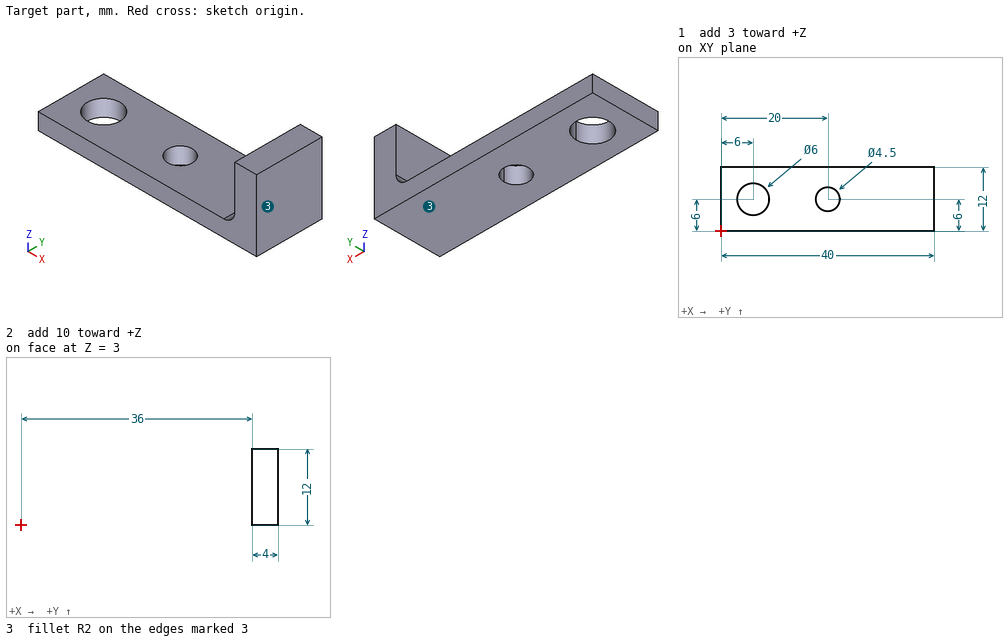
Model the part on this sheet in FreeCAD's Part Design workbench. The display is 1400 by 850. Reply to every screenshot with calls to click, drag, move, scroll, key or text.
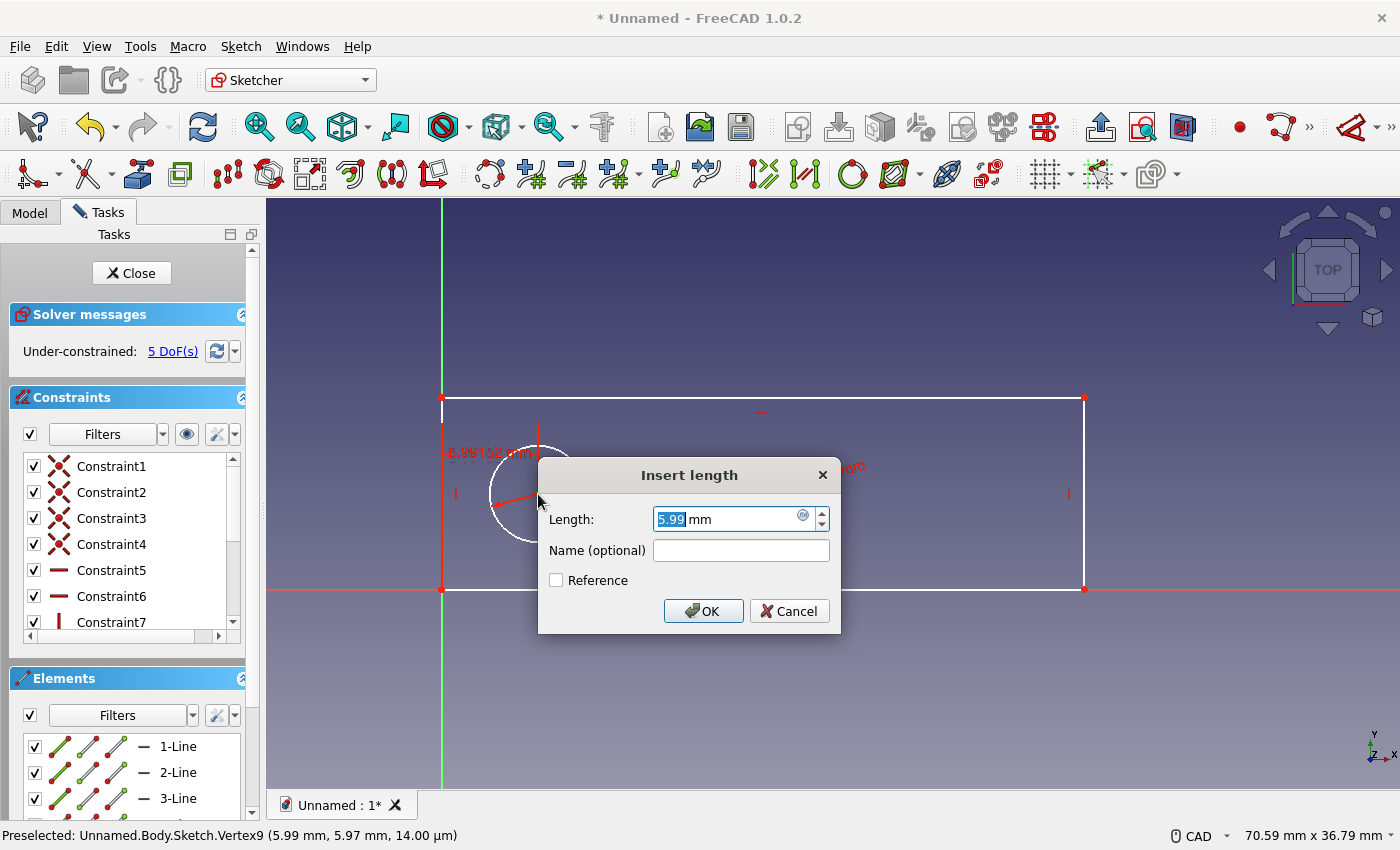
text(6)
key(Return)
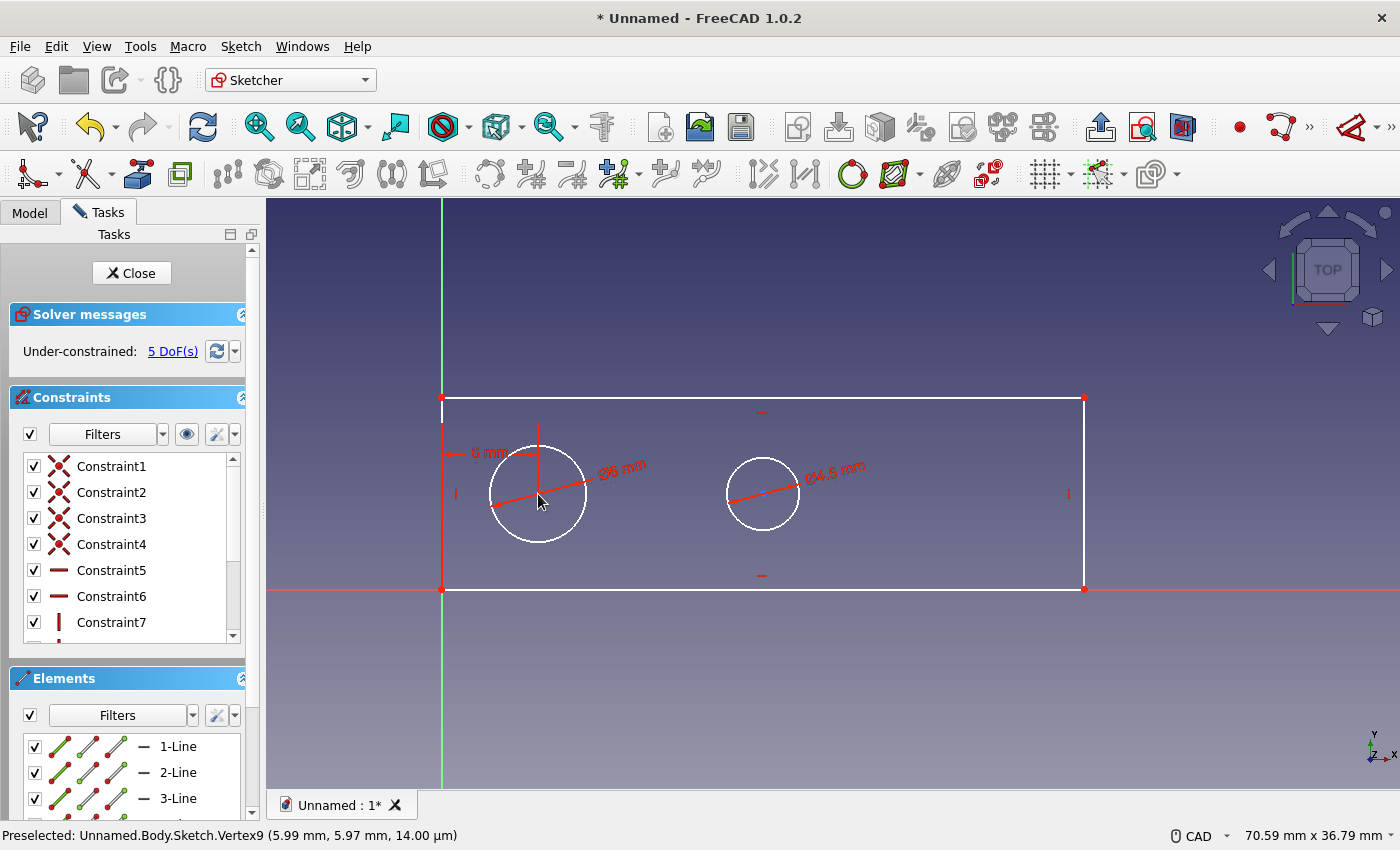
click(538, 494)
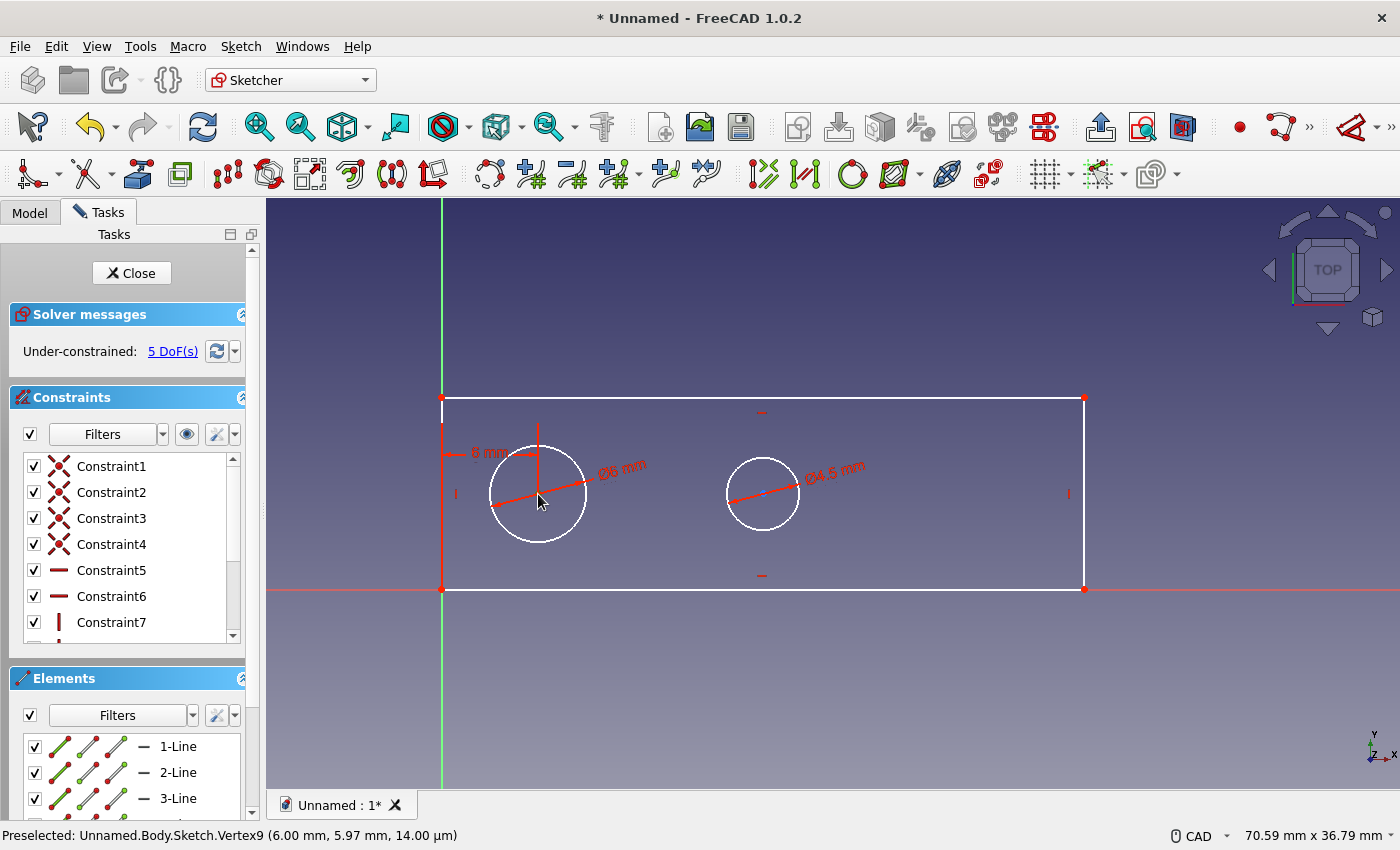
key(i)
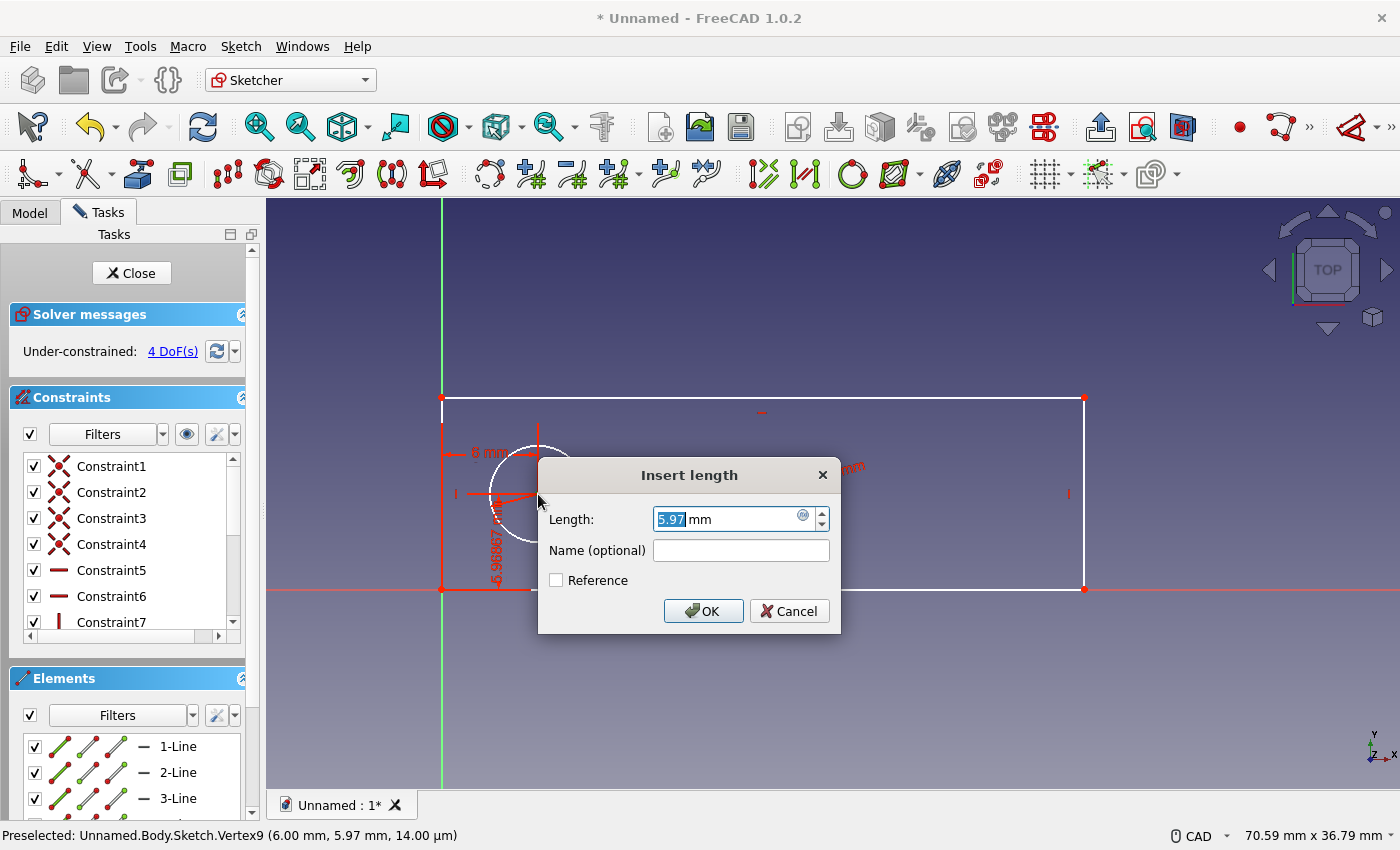
text(6)
key(Return)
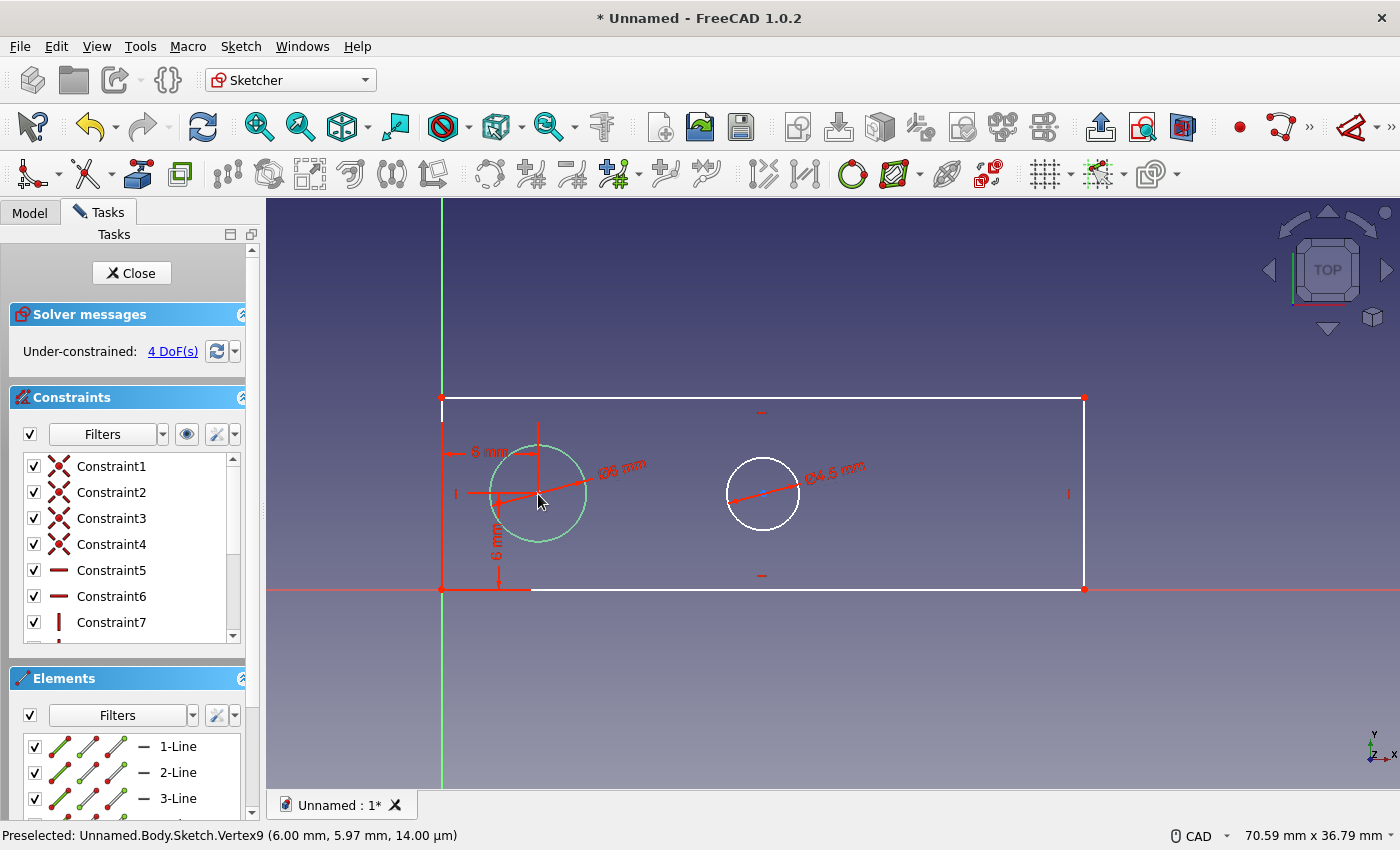
click(763, 494)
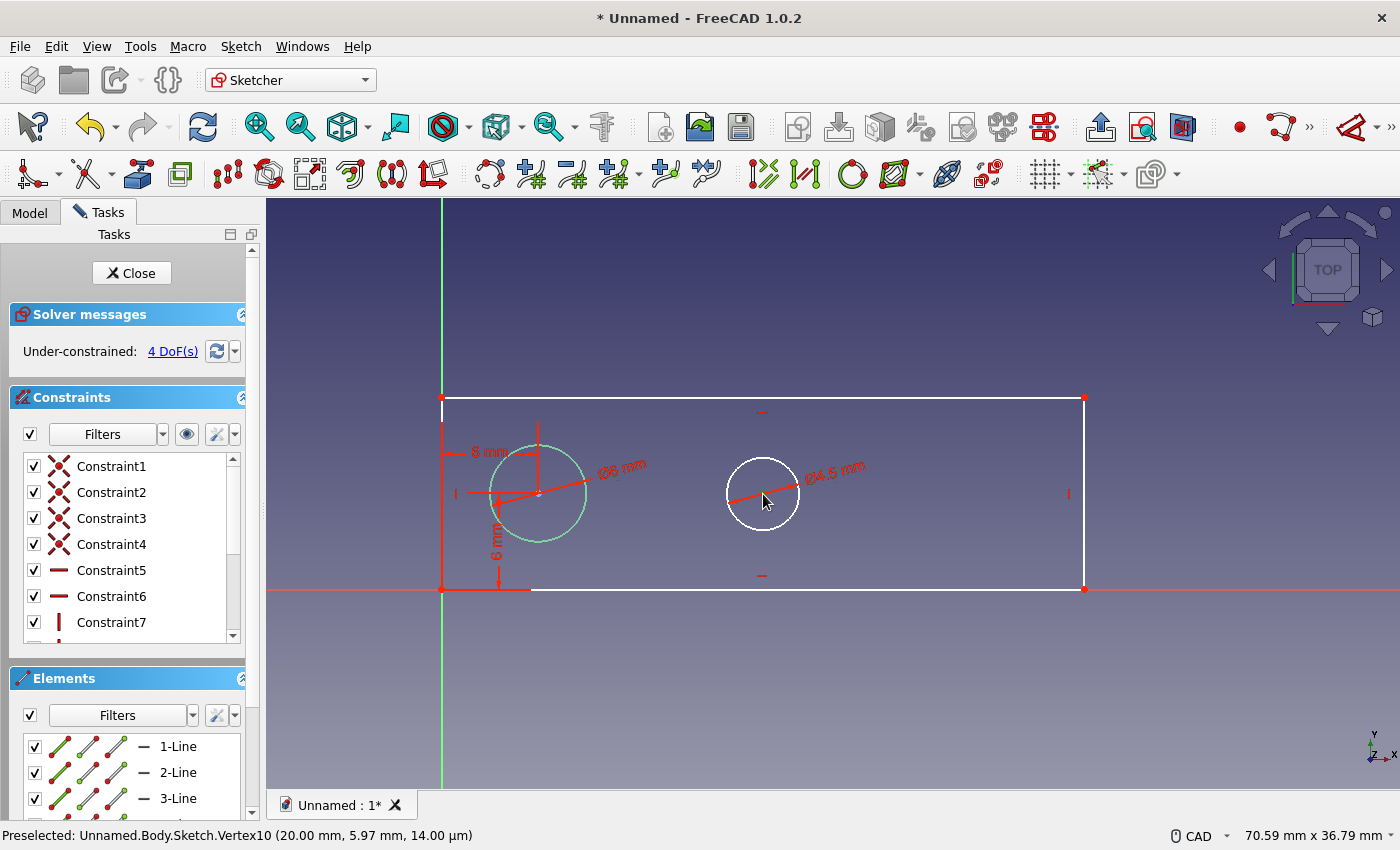
key(i)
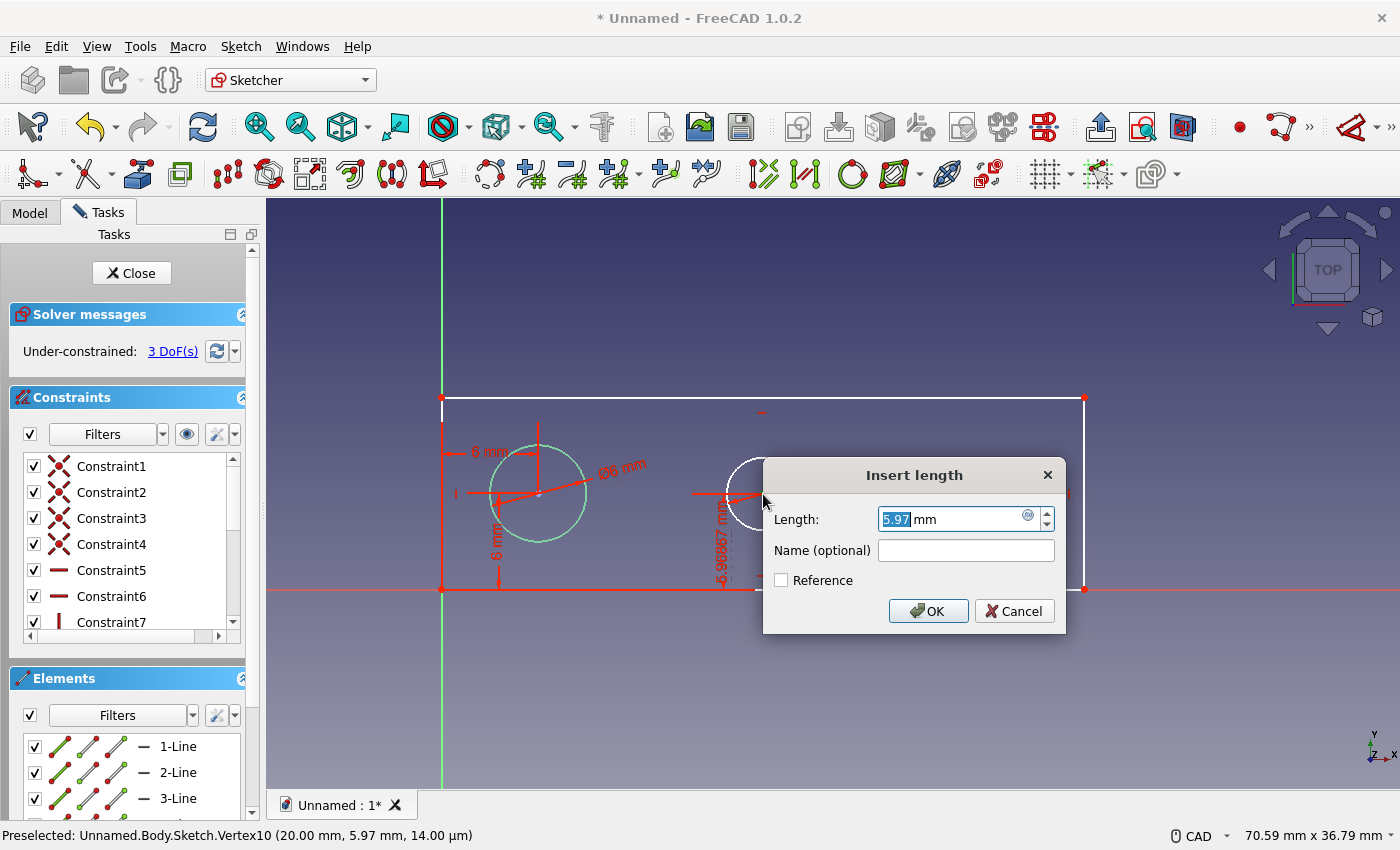
text(6)
key(Return)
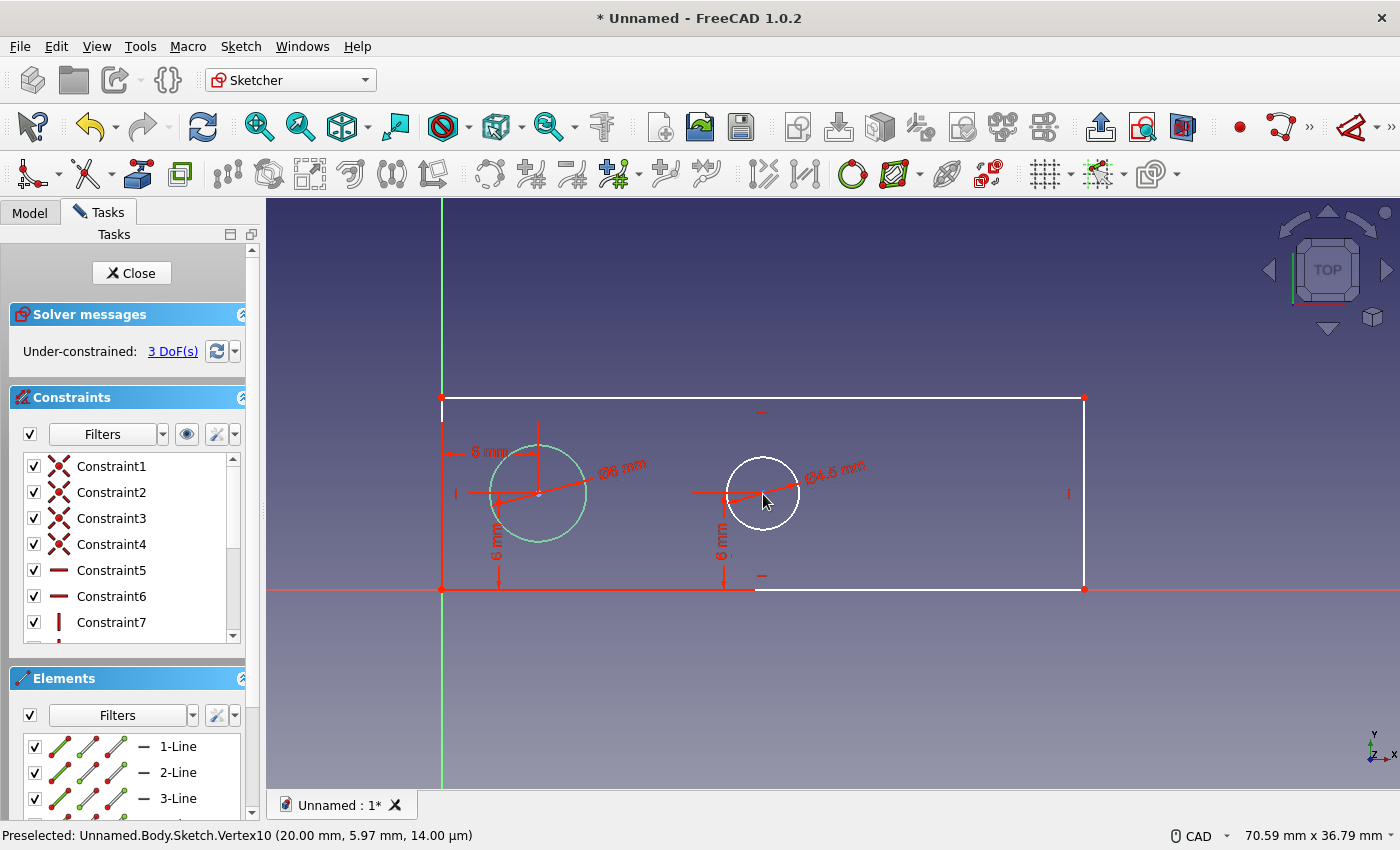
click(634, 590)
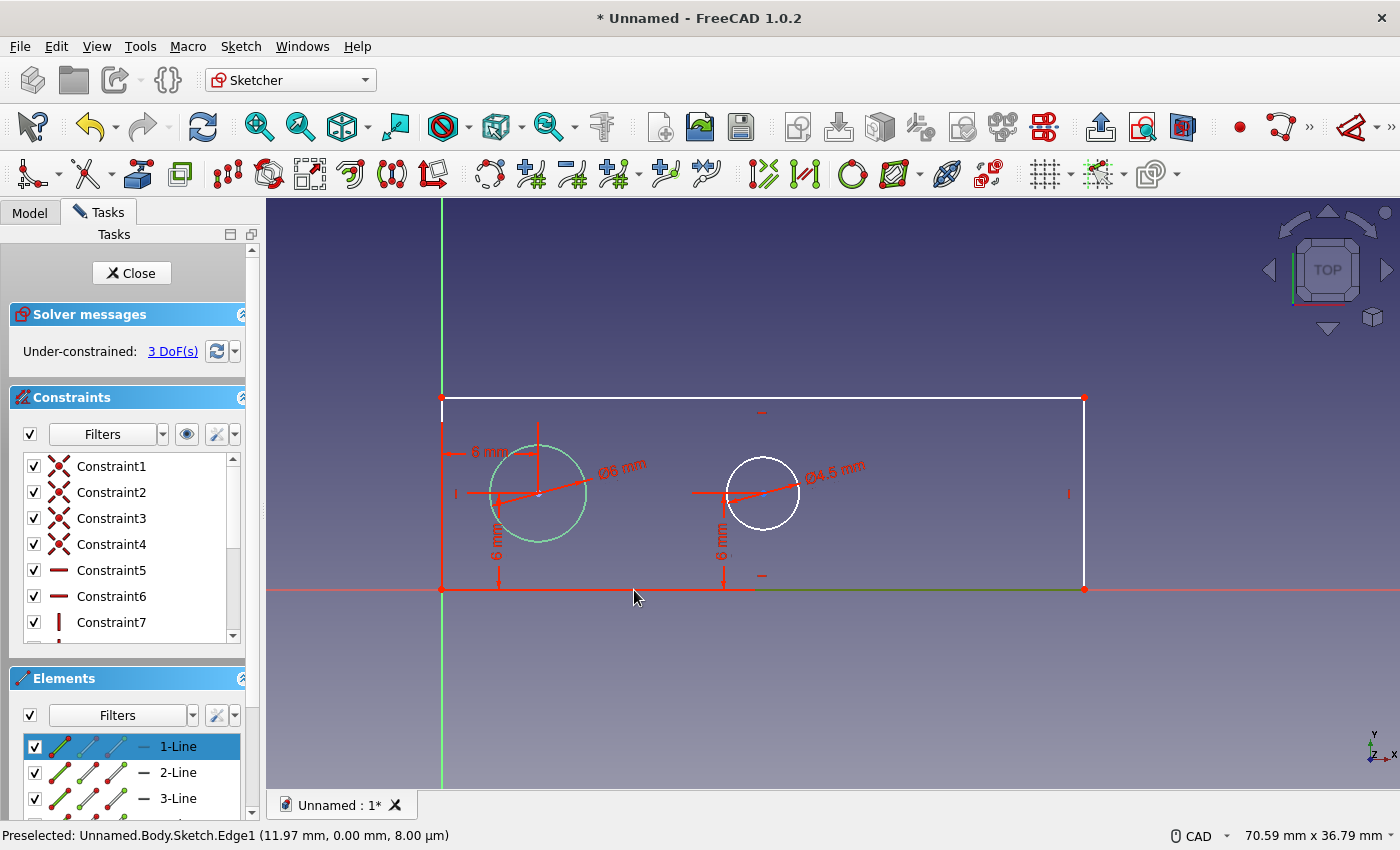
key(l)